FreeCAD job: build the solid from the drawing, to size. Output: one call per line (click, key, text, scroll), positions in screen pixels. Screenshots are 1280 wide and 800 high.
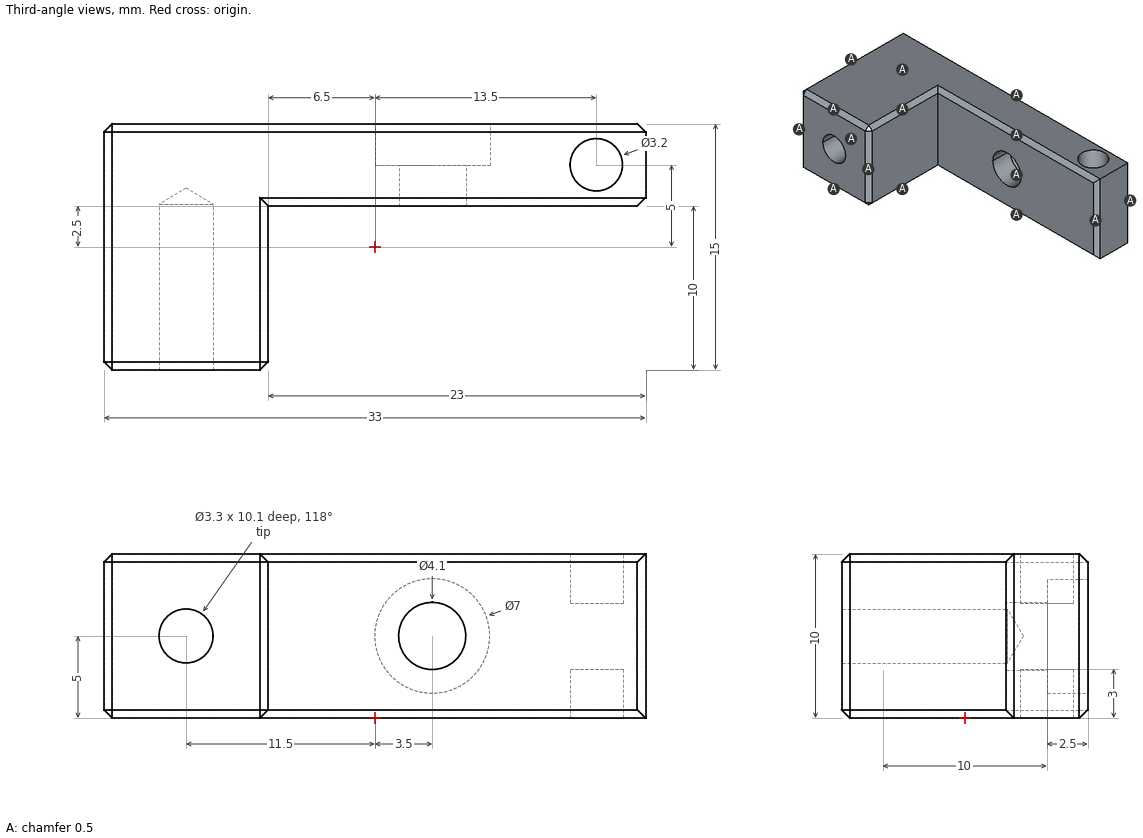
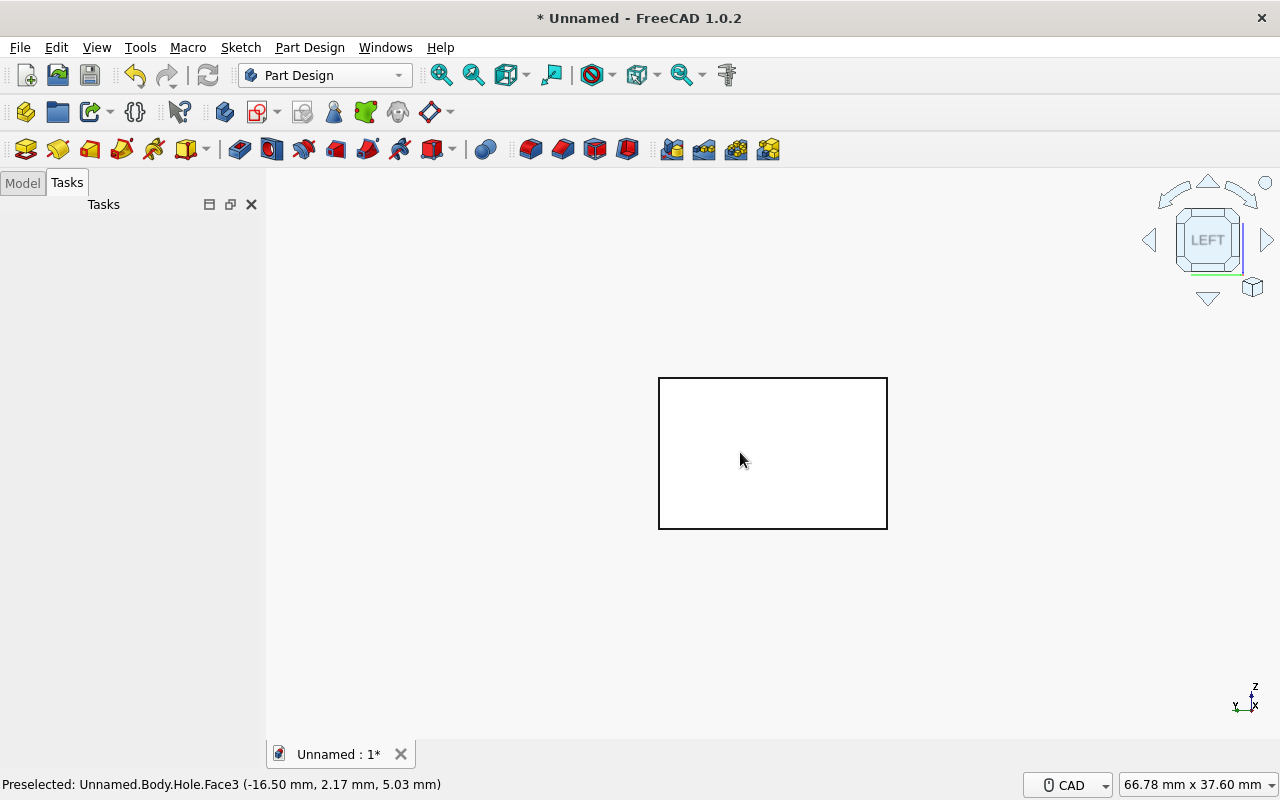
click(564, 150)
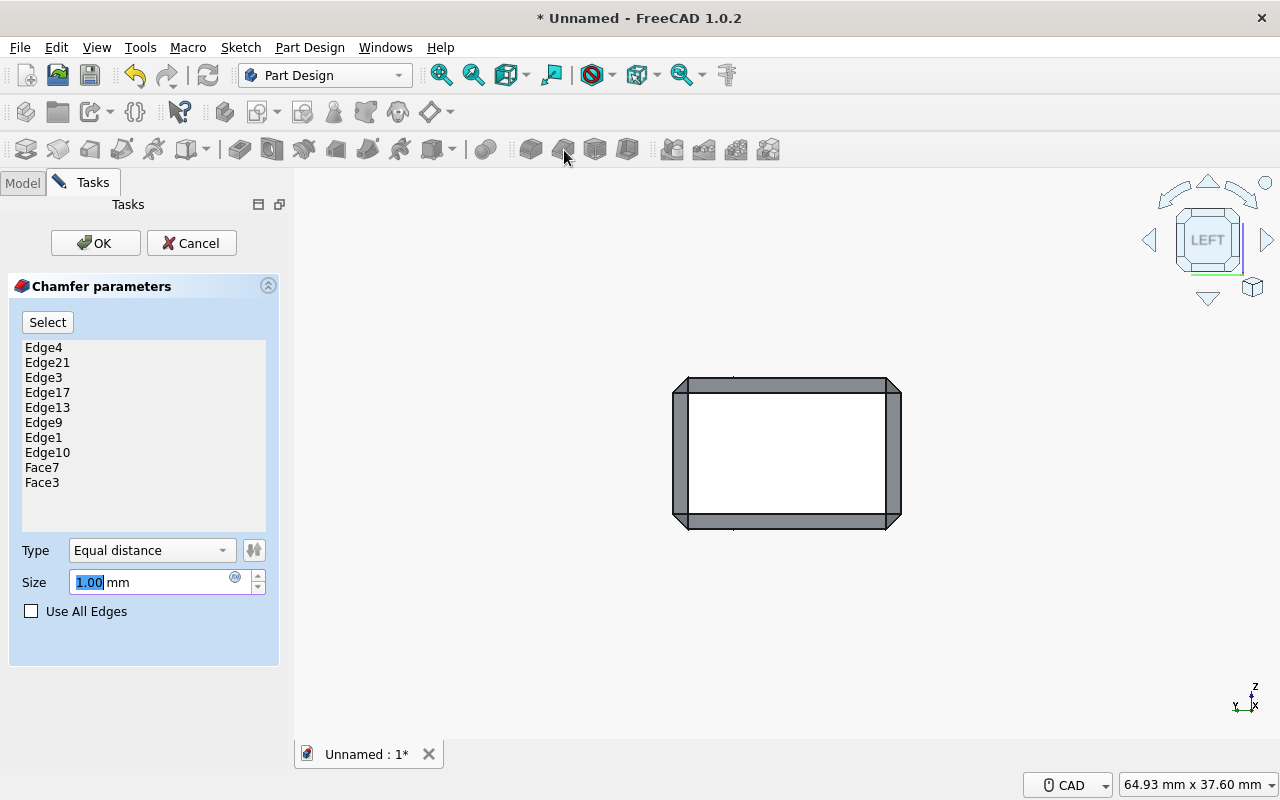
text(0.5)
key(Tab)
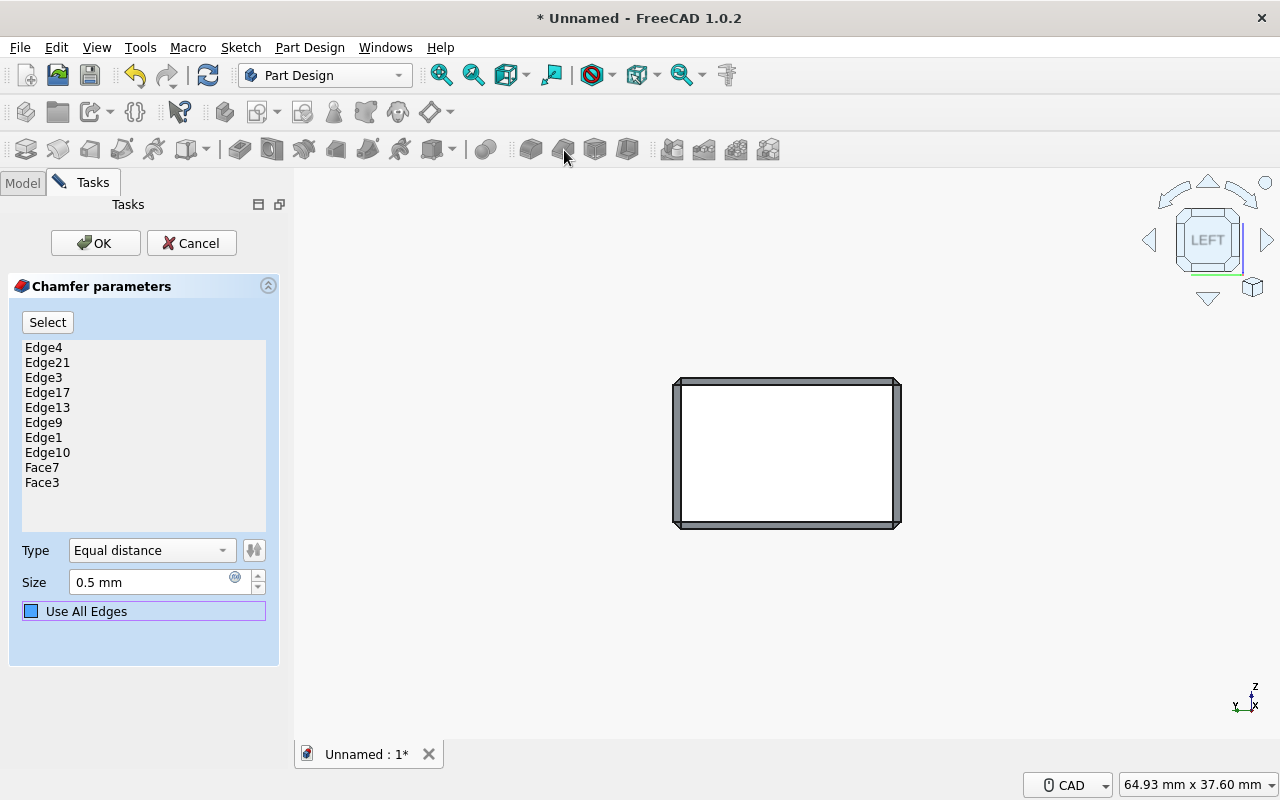
click(96, 243)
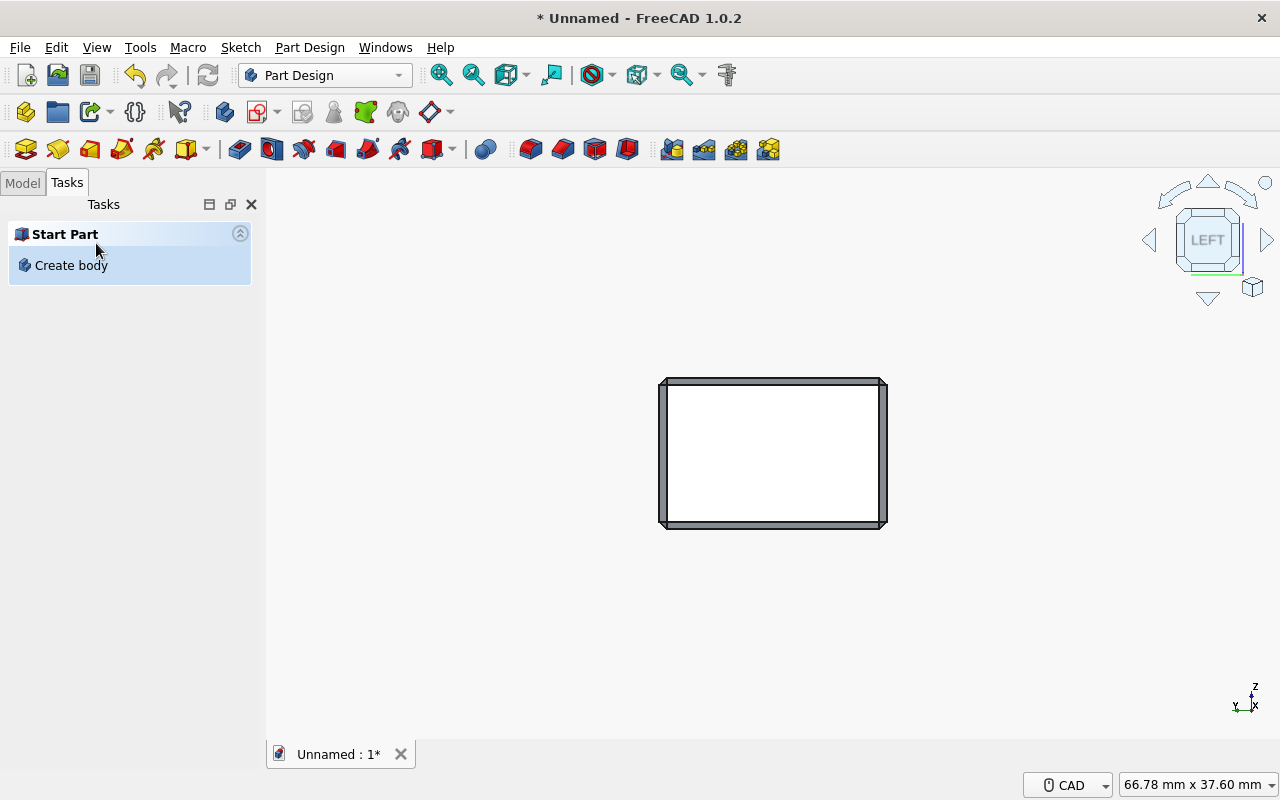
click(442, 76)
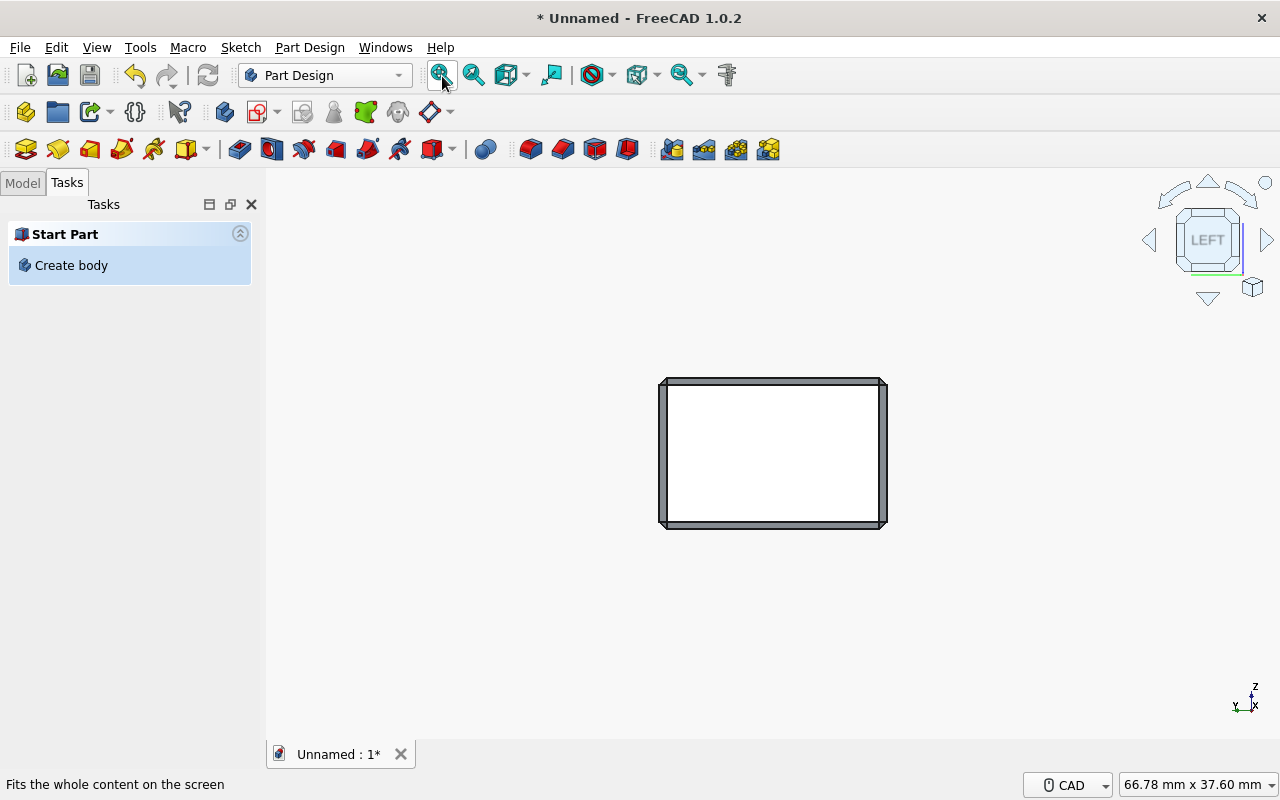
key(4)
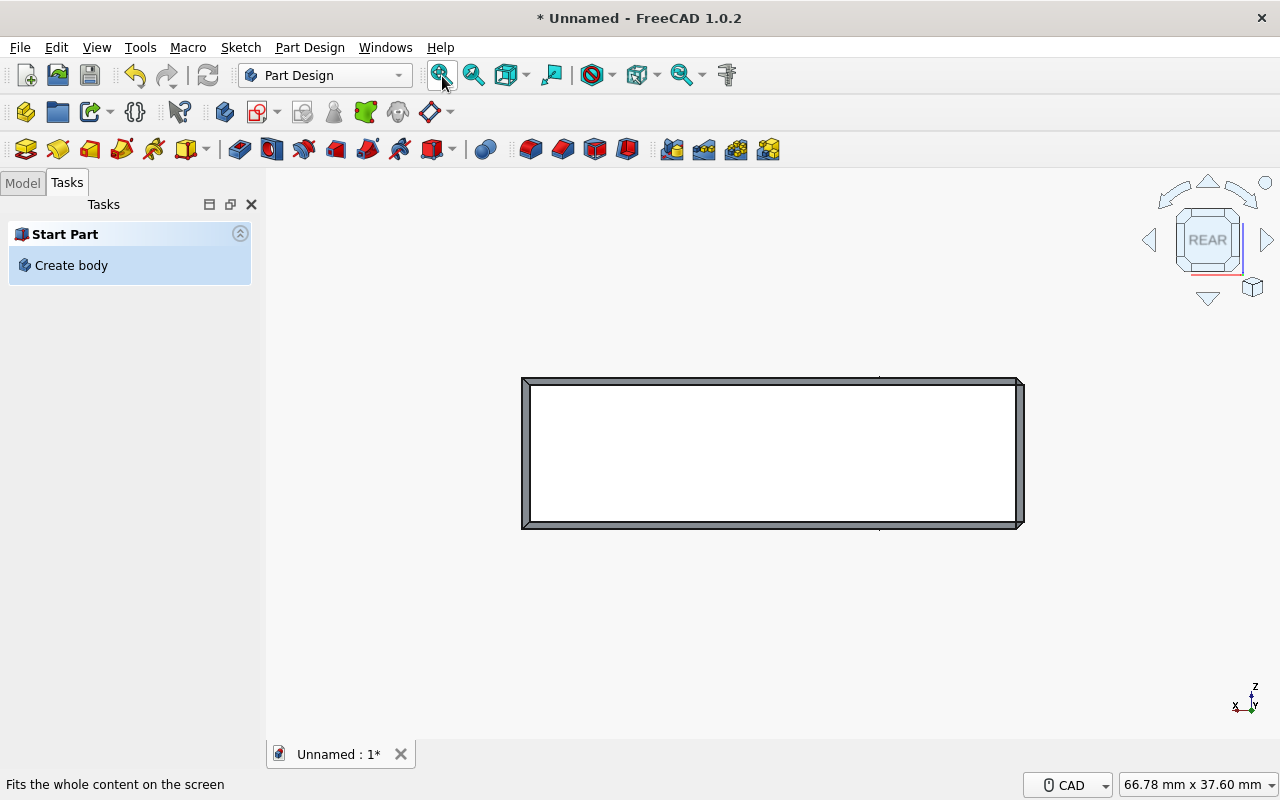
click(634, 452)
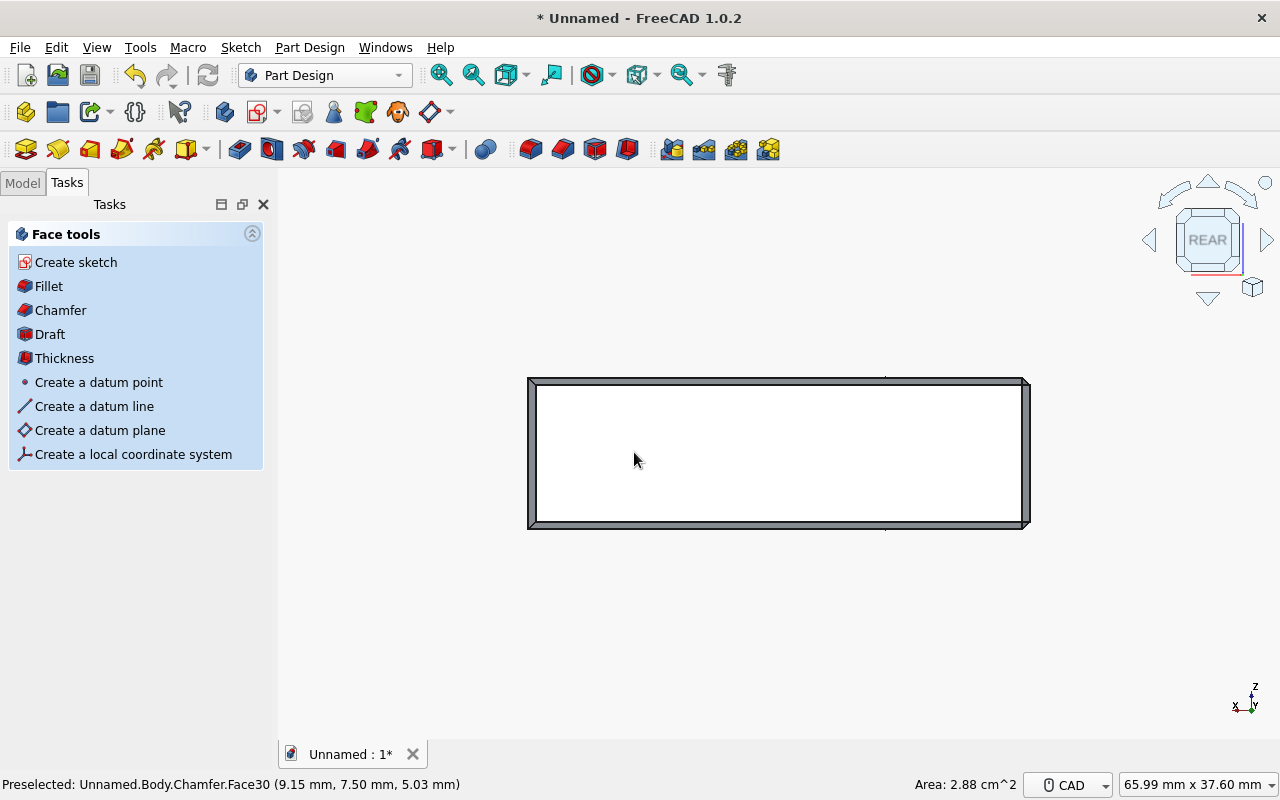
click(258, 112)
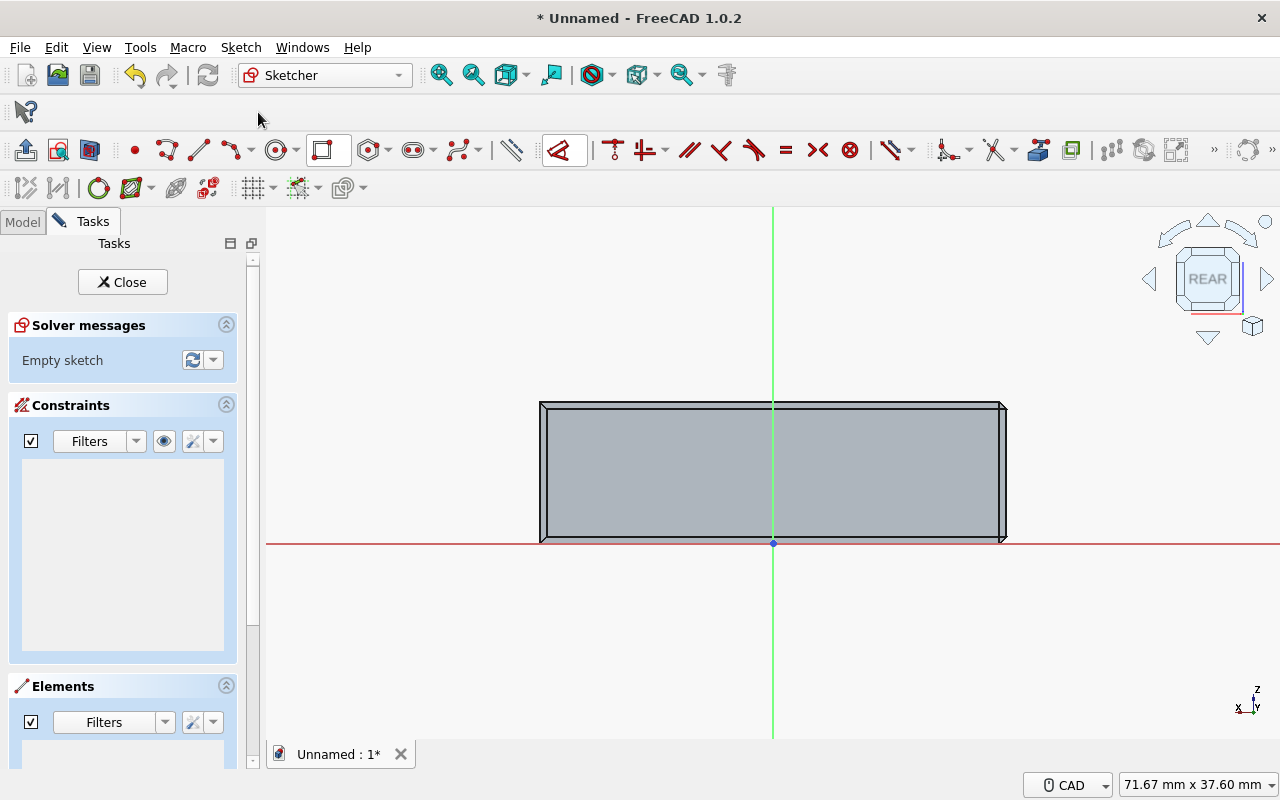
scroll(735, 490, up, 5)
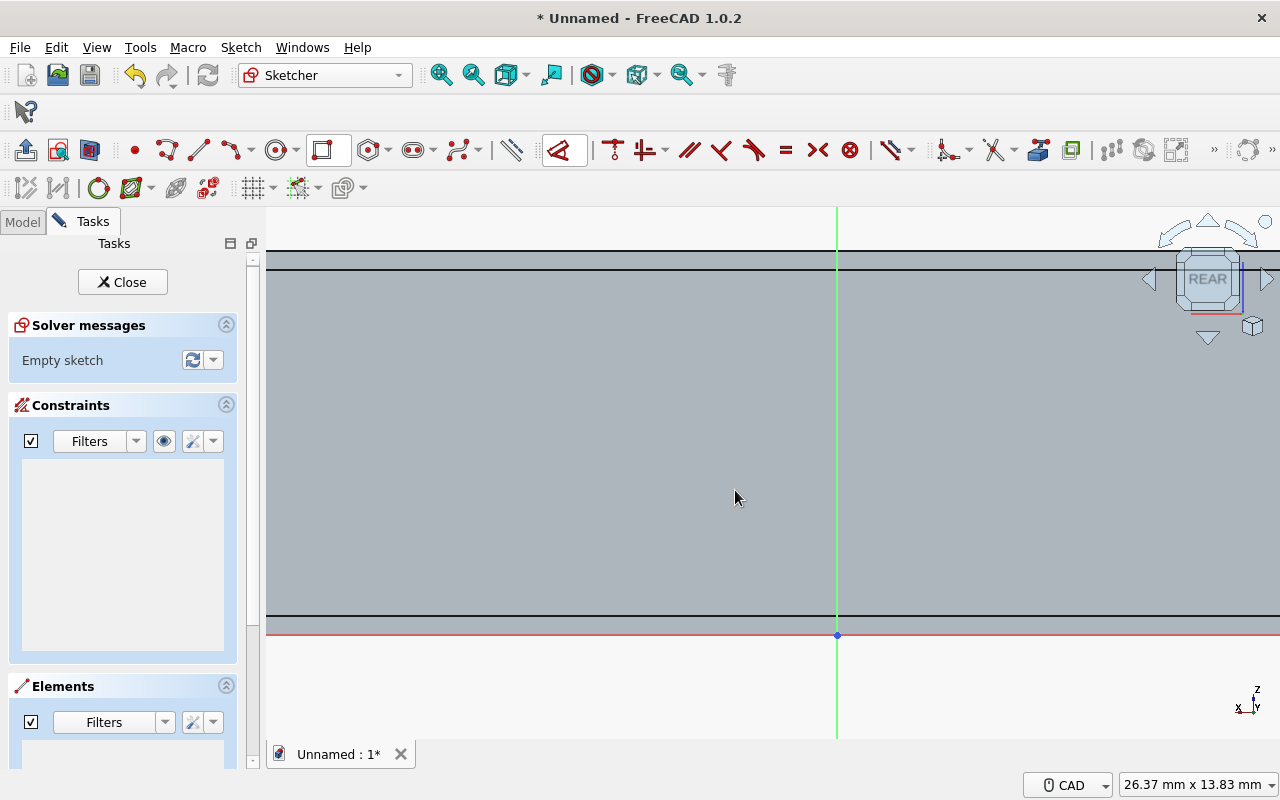
click(276, 150)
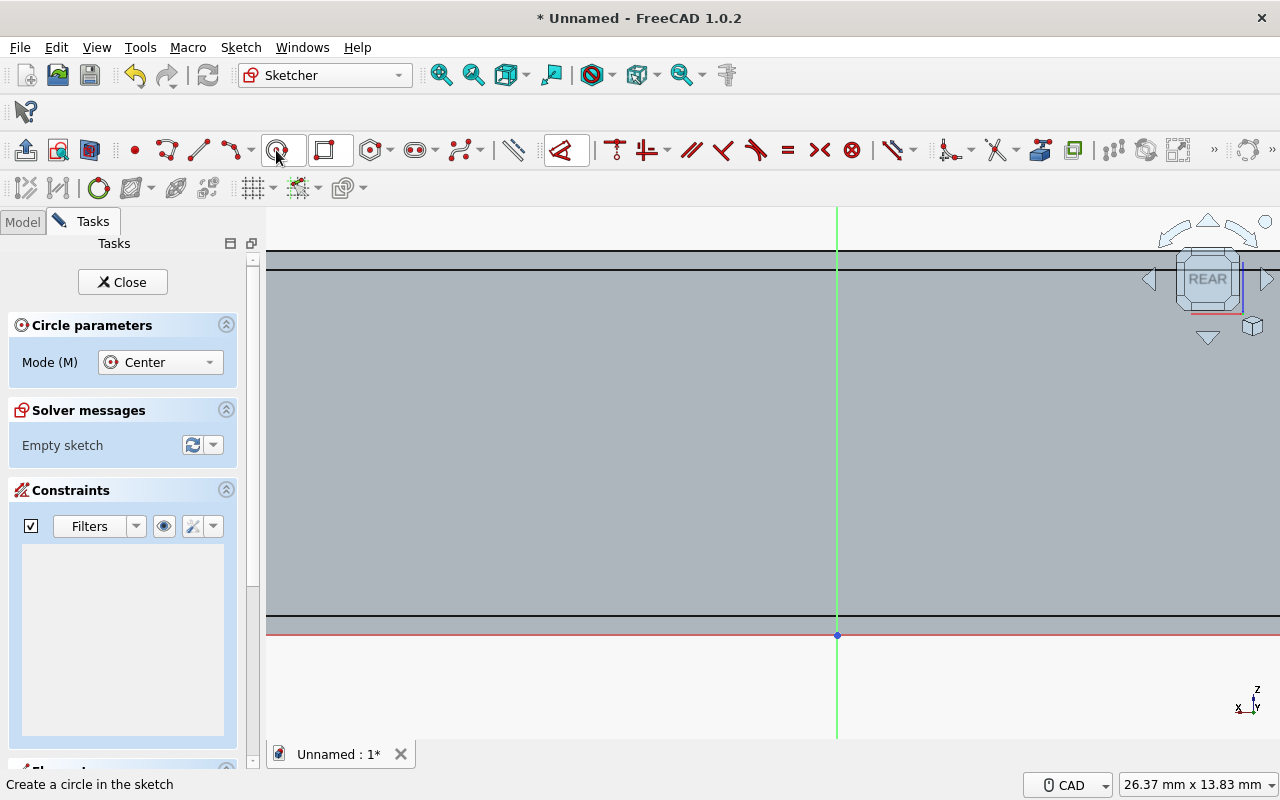
click(703, 443)
move(798, 348)